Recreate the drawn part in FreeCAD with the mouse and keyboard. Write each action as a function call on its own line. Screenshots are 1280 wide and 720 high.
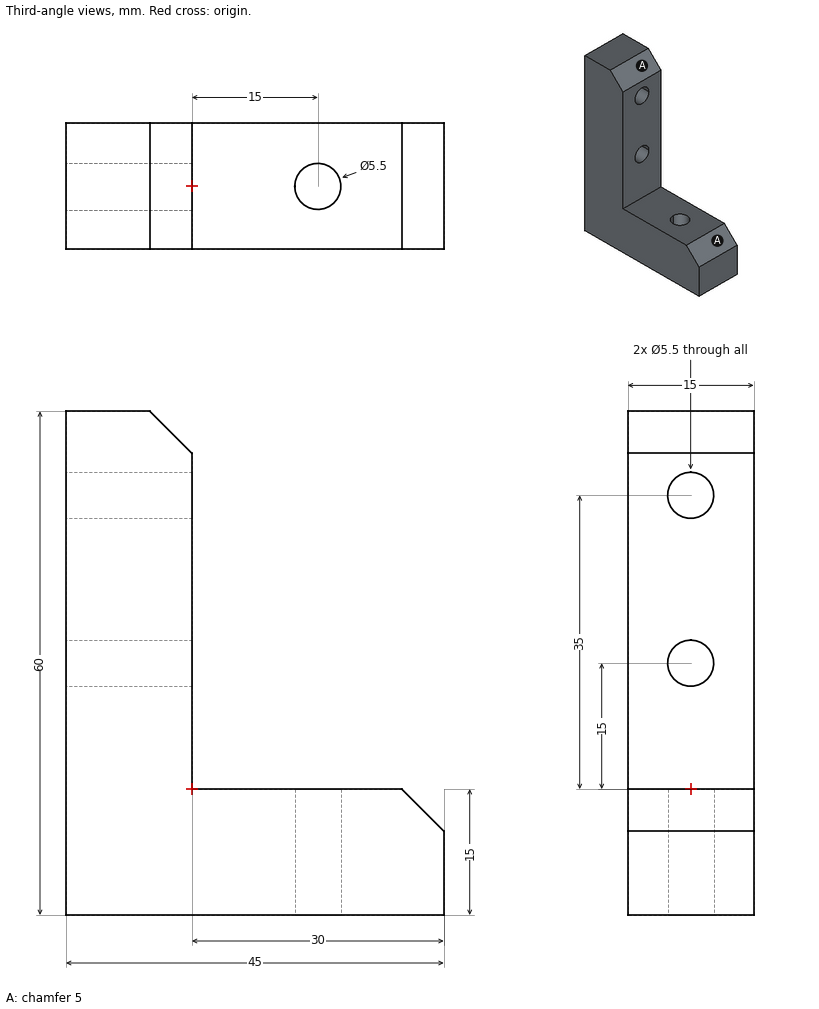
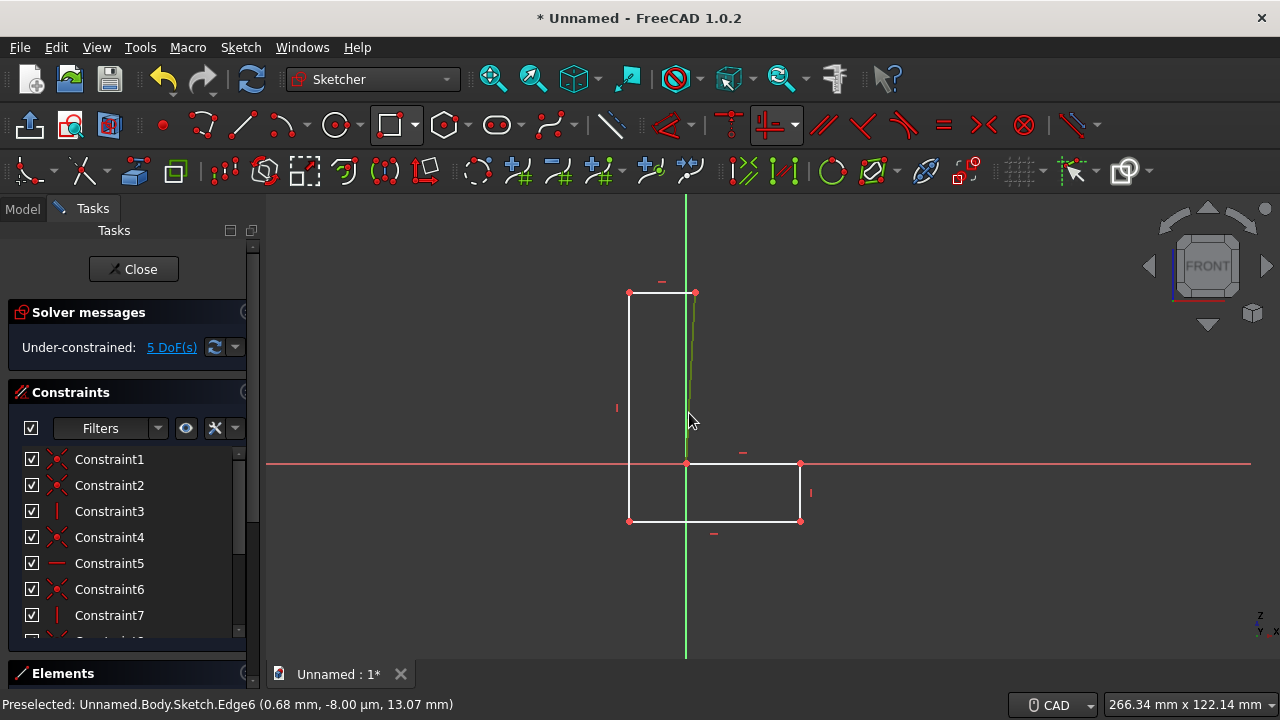
key(v)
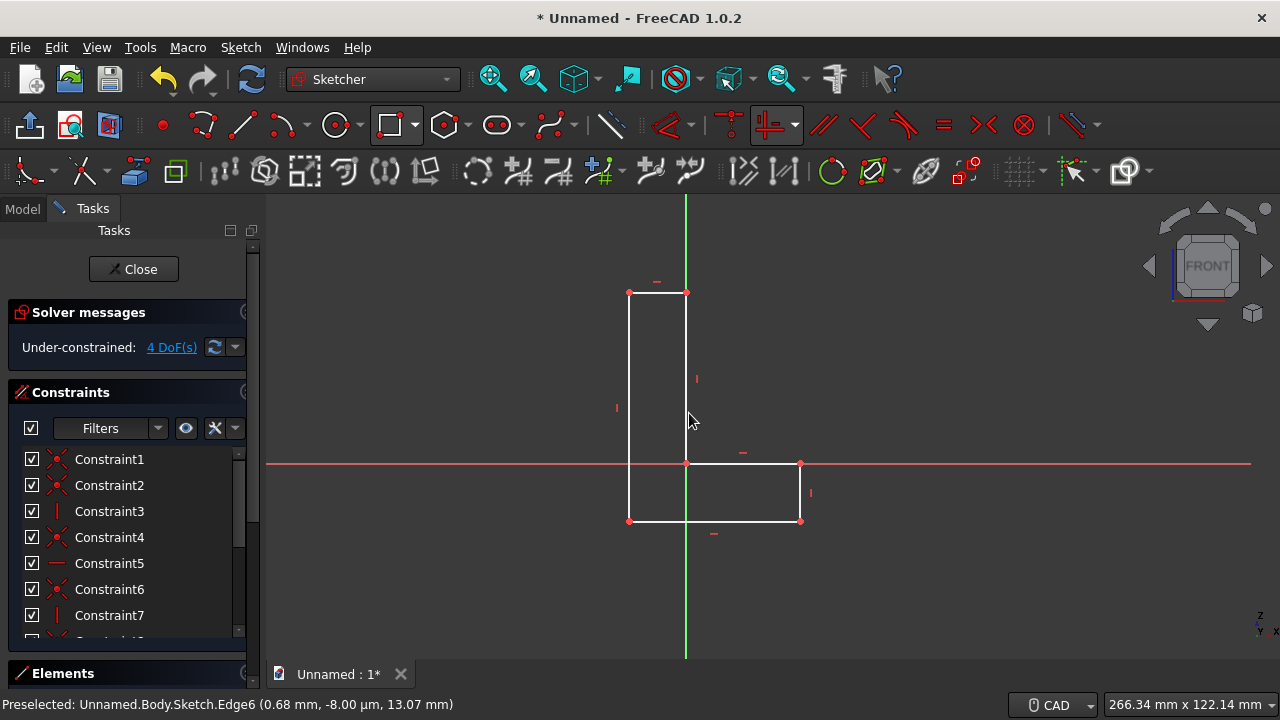
key(d)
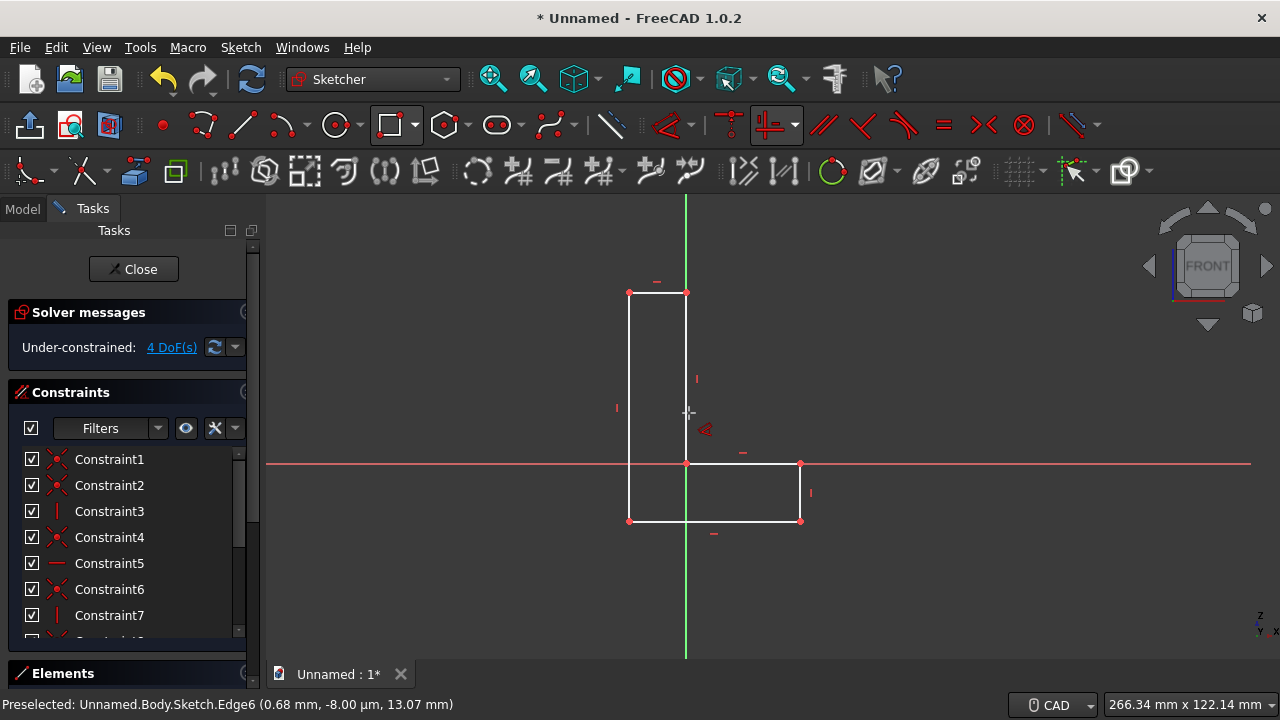
click(720, 464)
click(743, 498)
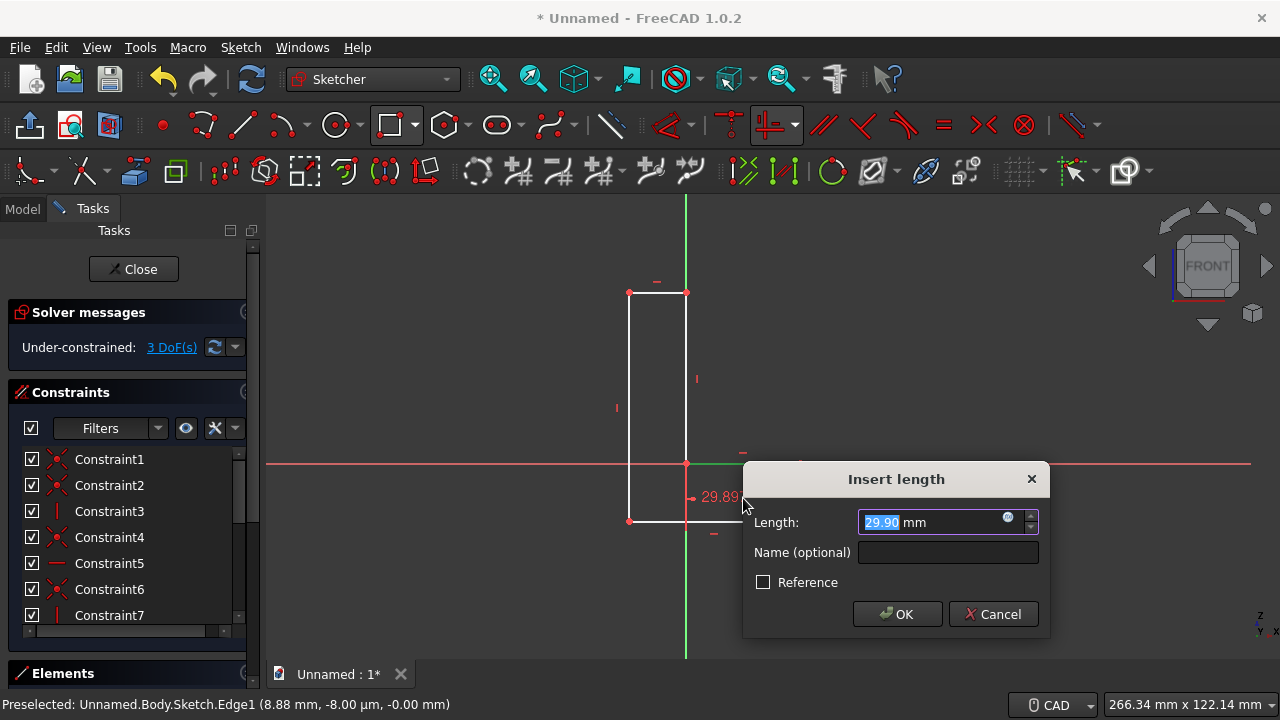
text(30)
key(Return)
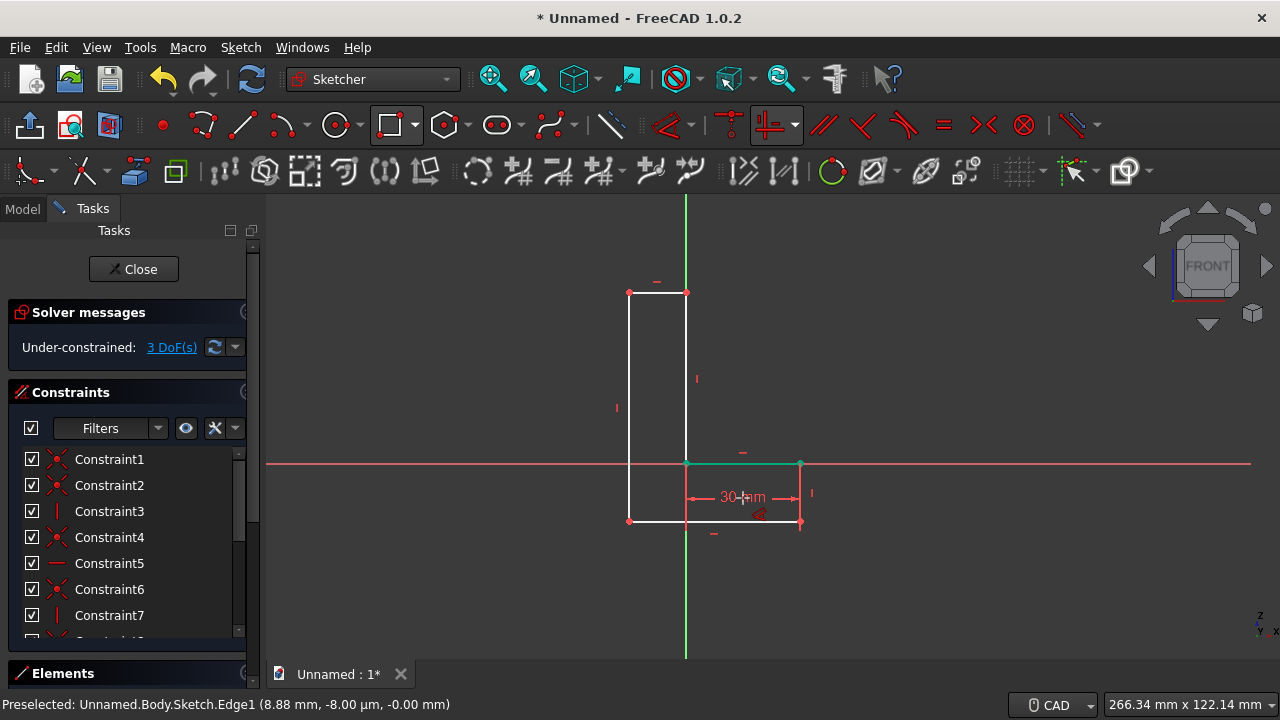
click(800, 481)
click(834, 493)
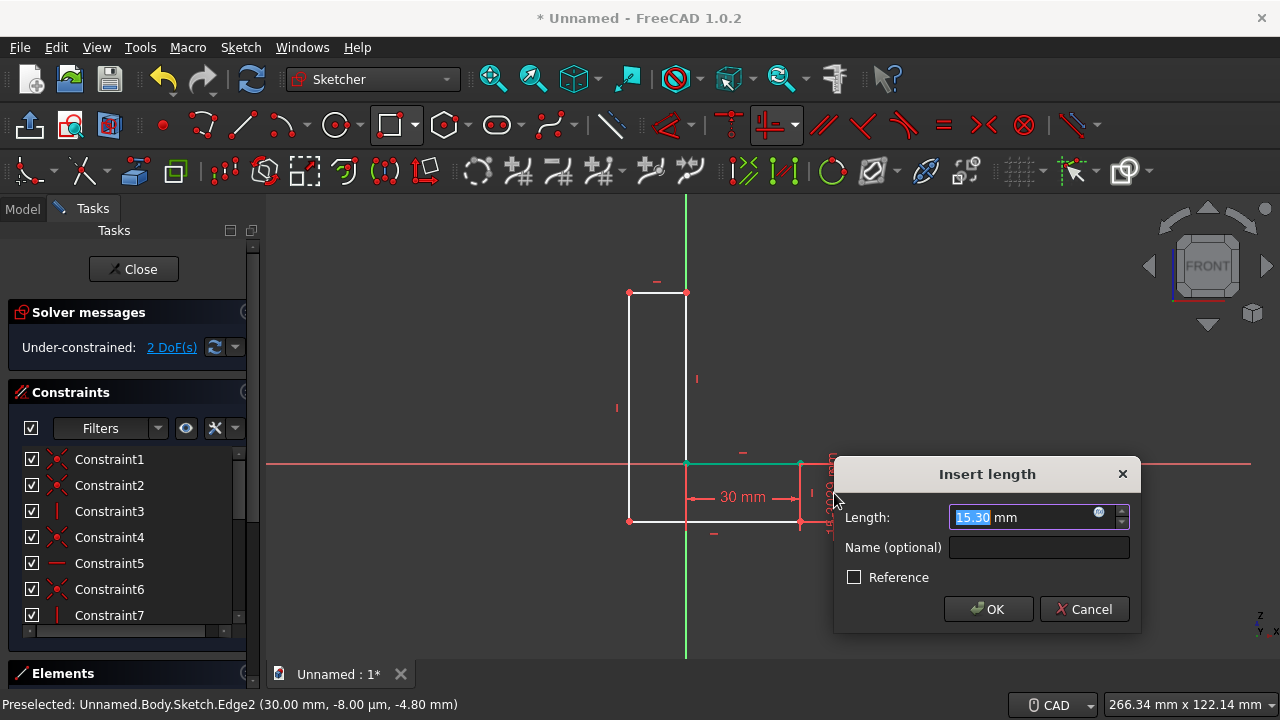
text(15)
key(Return)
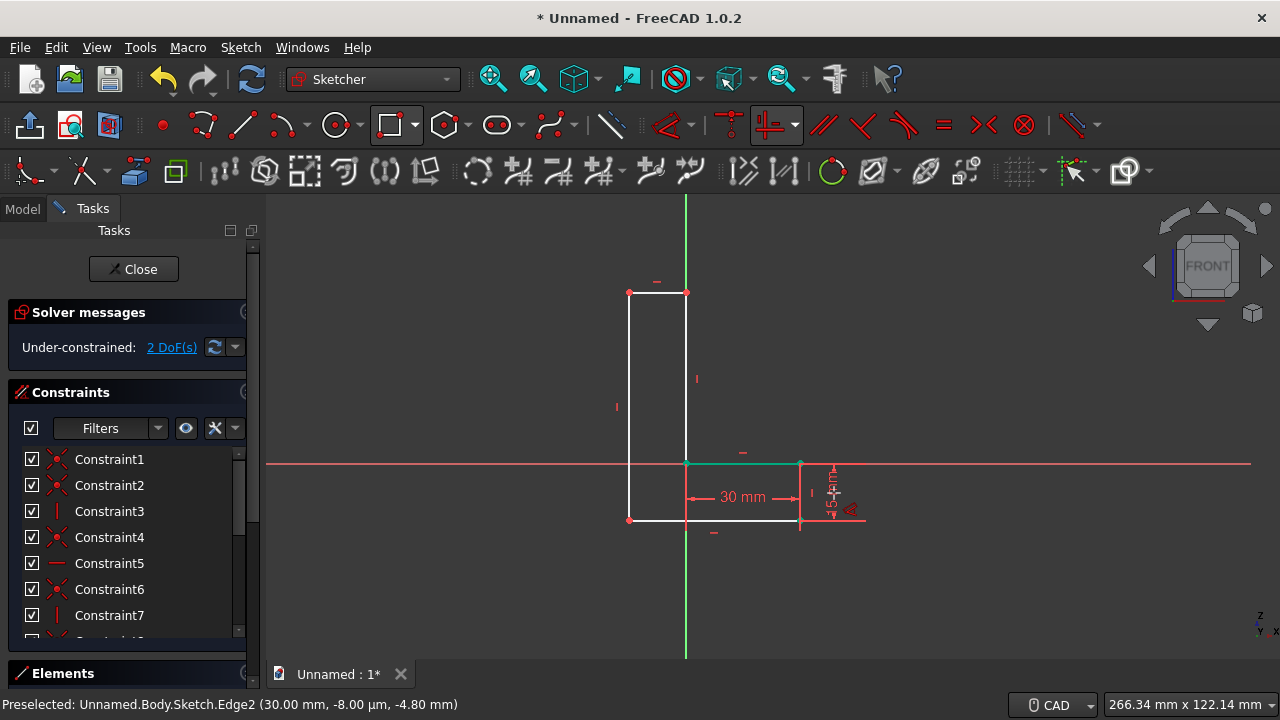
click(749, 521)
click(715, 555)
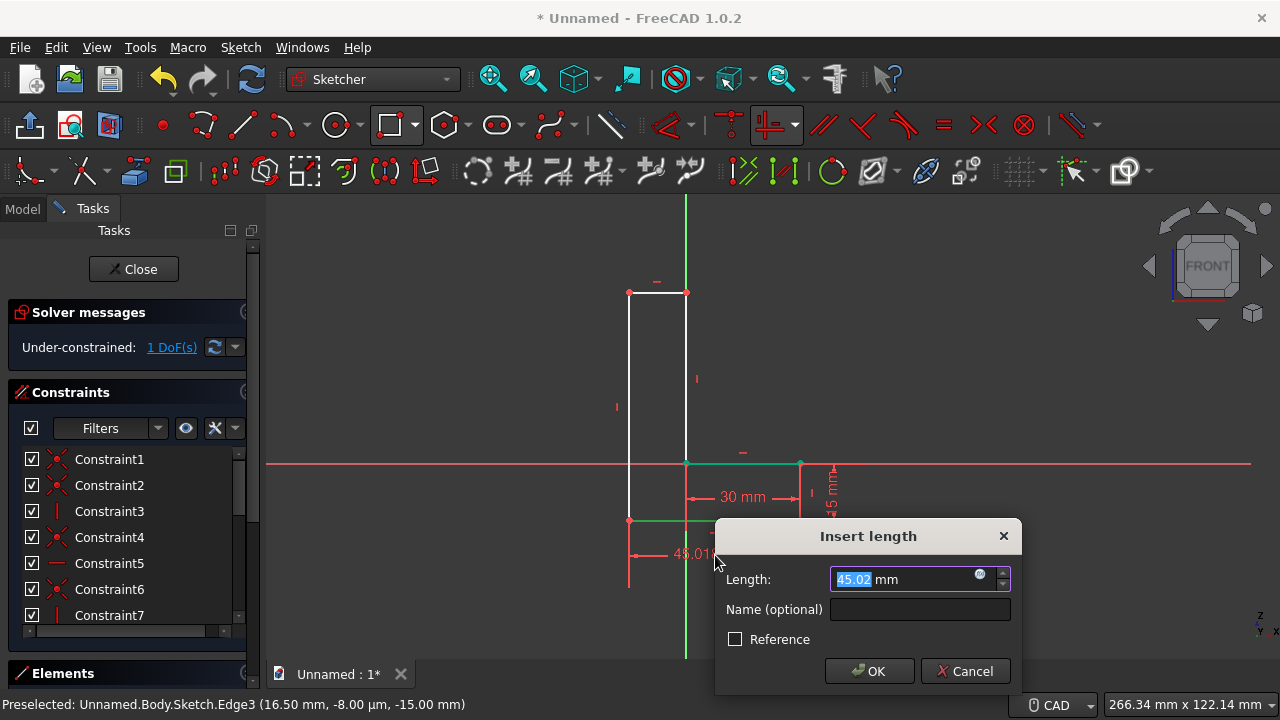
text(45)
key(Return)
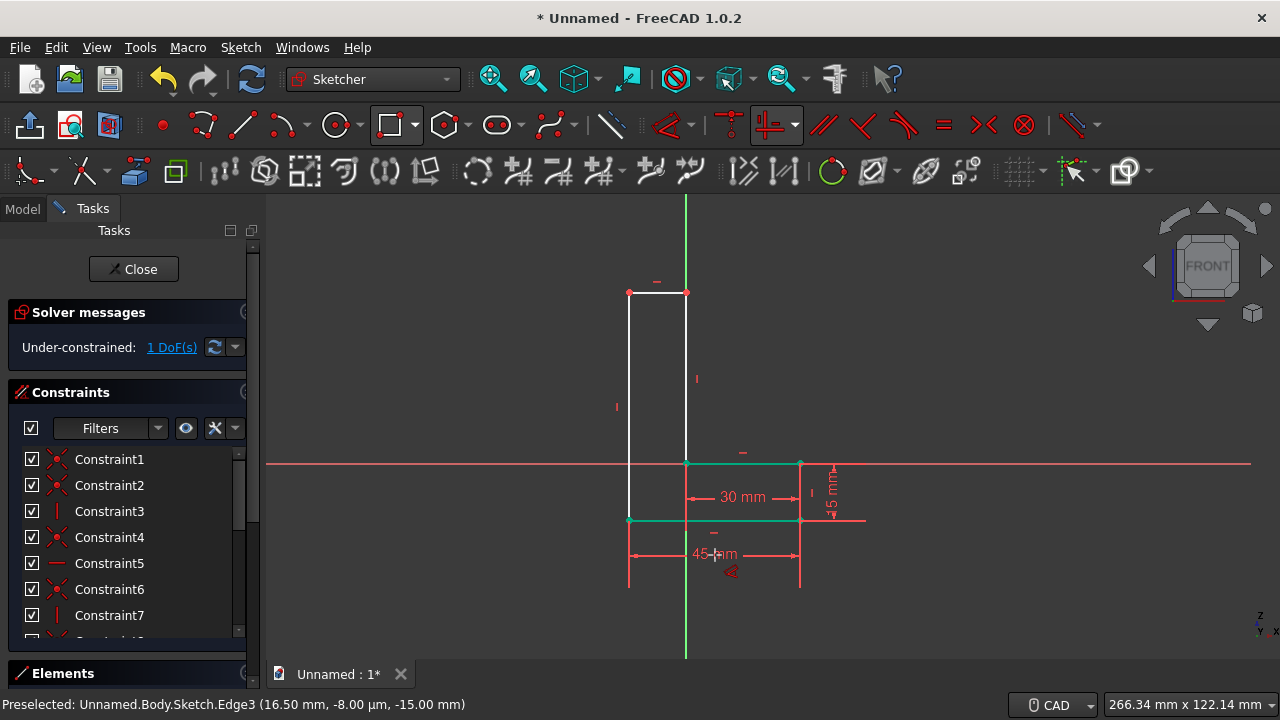
scroll(629, 452, up, 2)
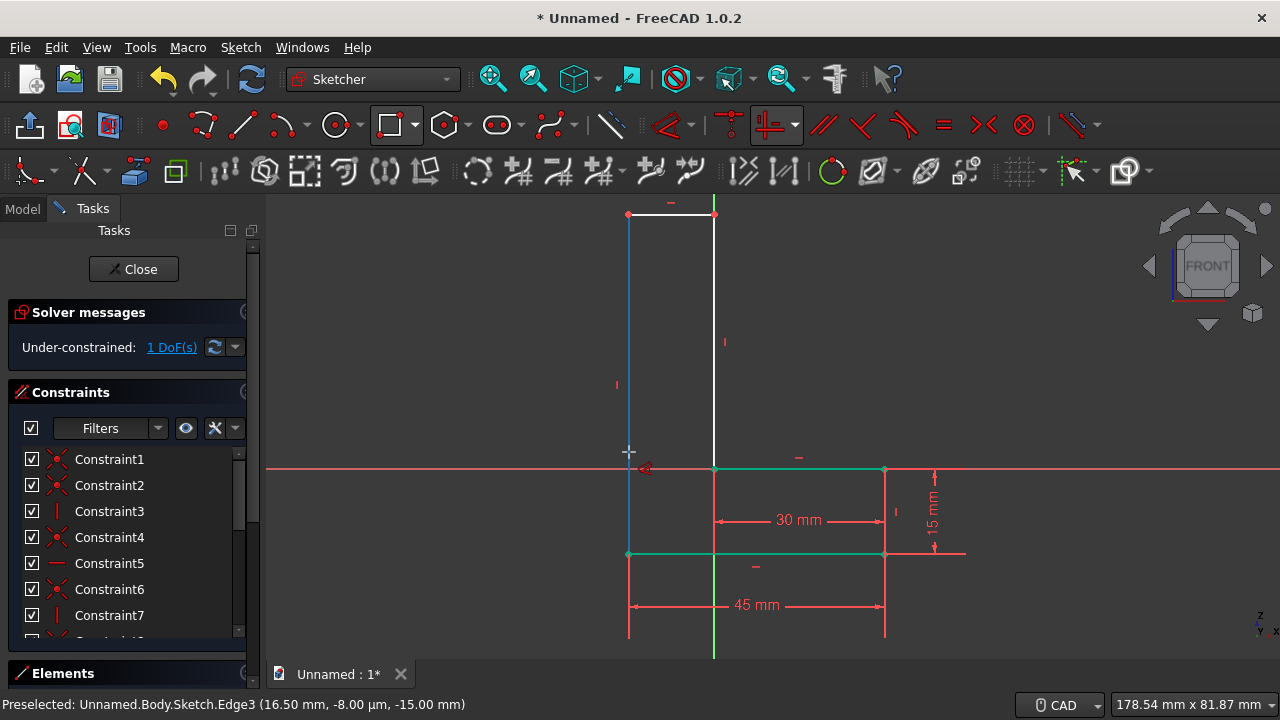
click(629, 452)
click(595, 388)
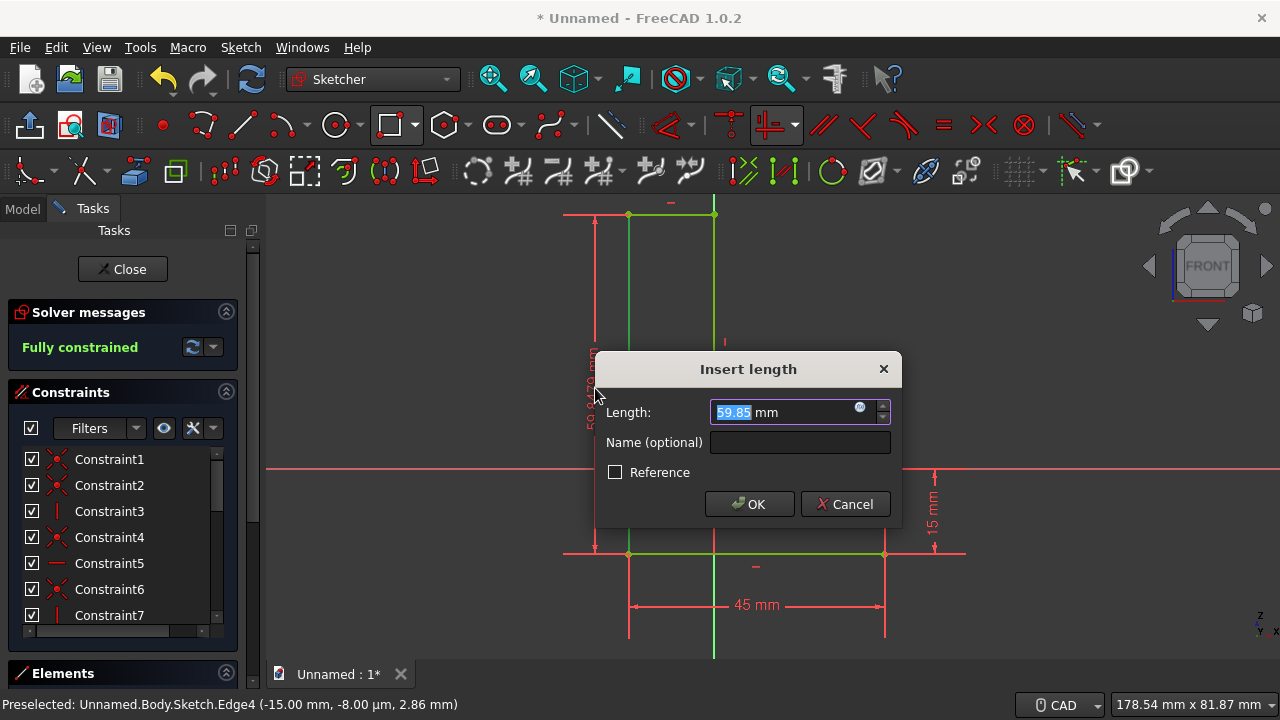
text(60)
key(Return)
key(Escape)